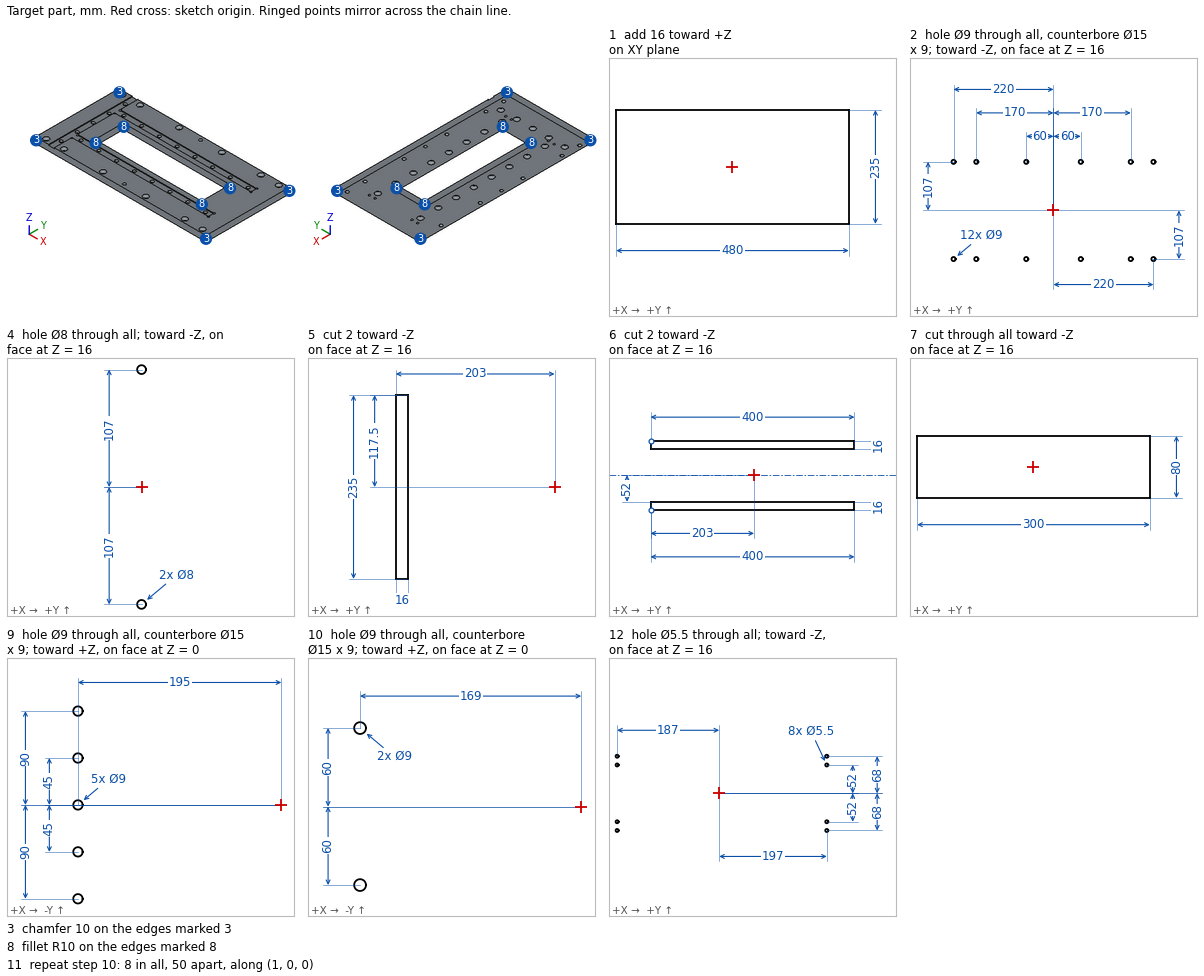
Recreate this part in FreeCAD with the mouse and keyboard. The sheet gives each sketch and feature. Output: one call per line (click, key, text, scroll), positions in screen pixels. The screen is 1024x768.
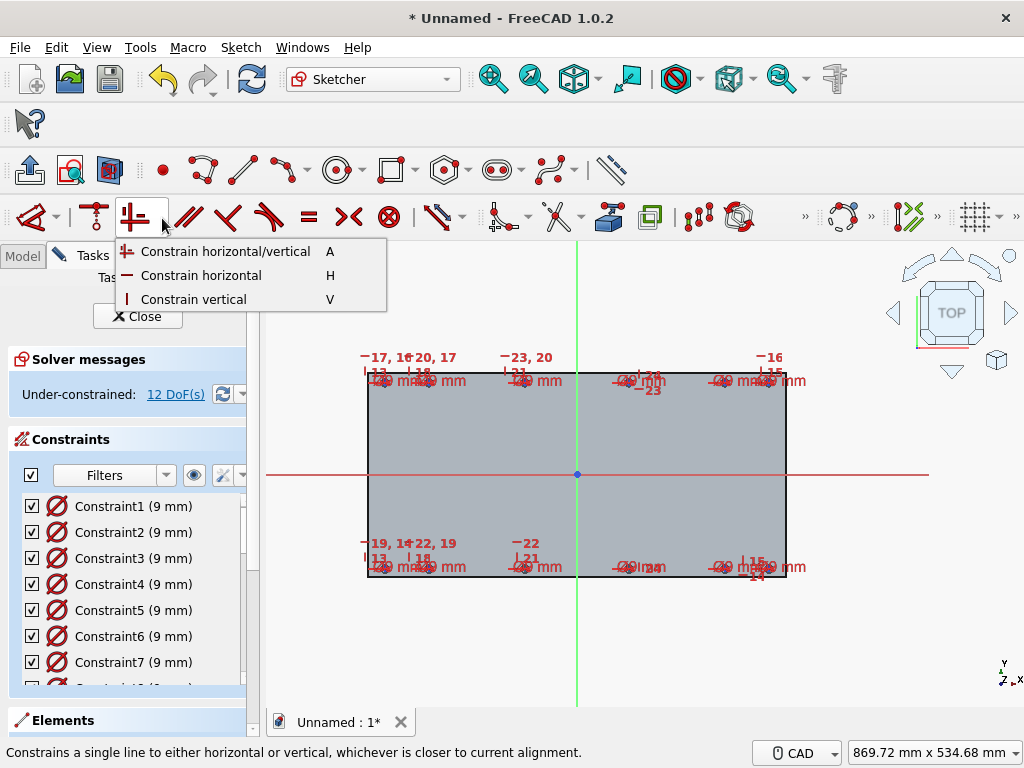
click(251, 275)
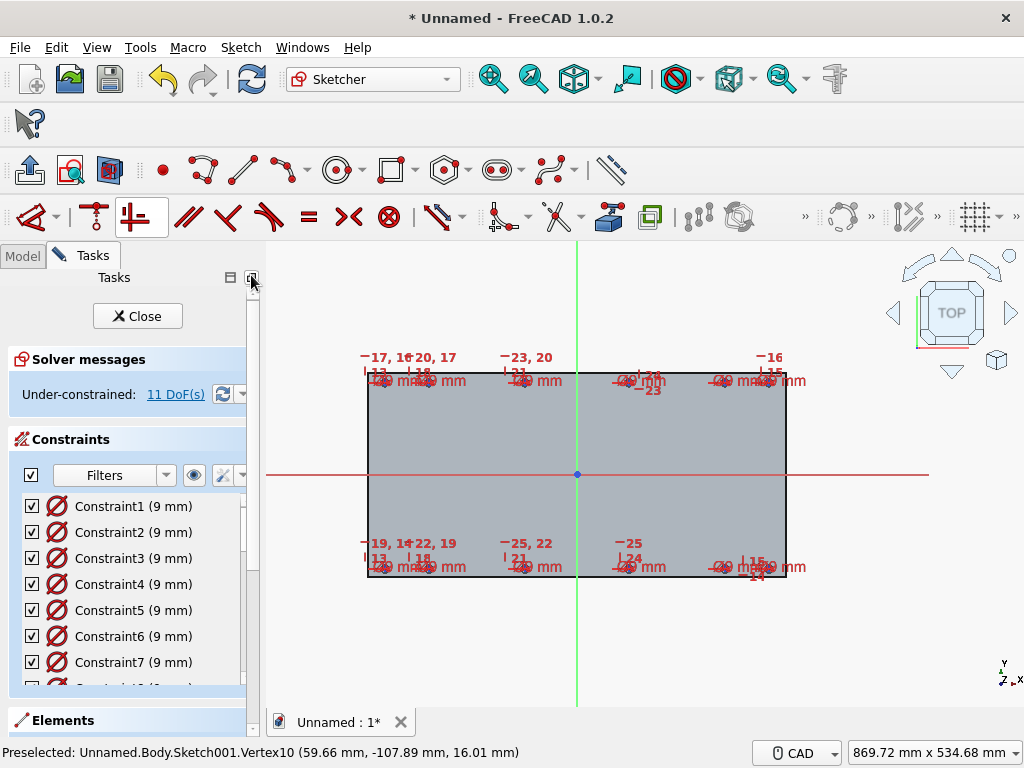
click(769, 383)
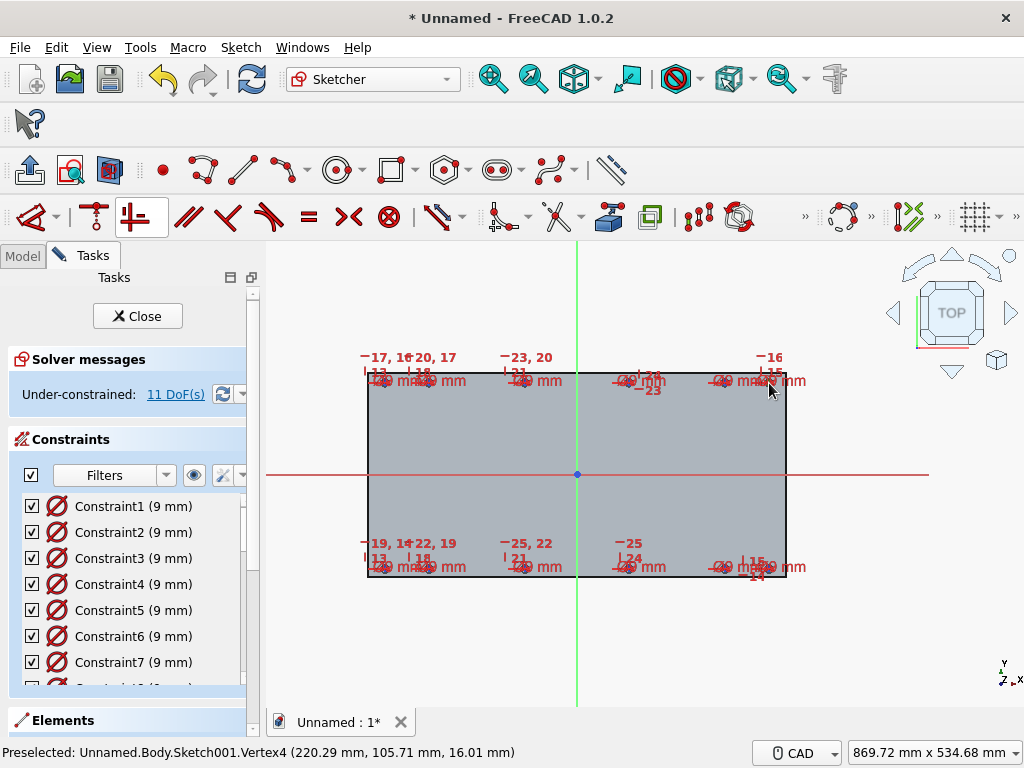
click(725, 383)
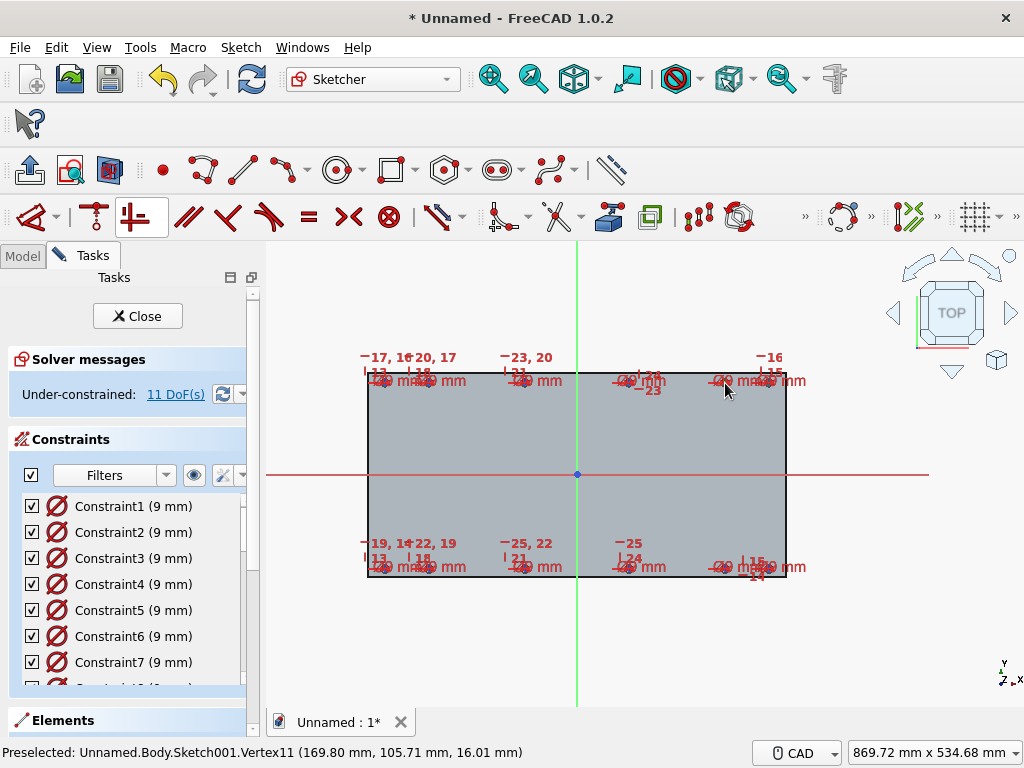
click(162, 218)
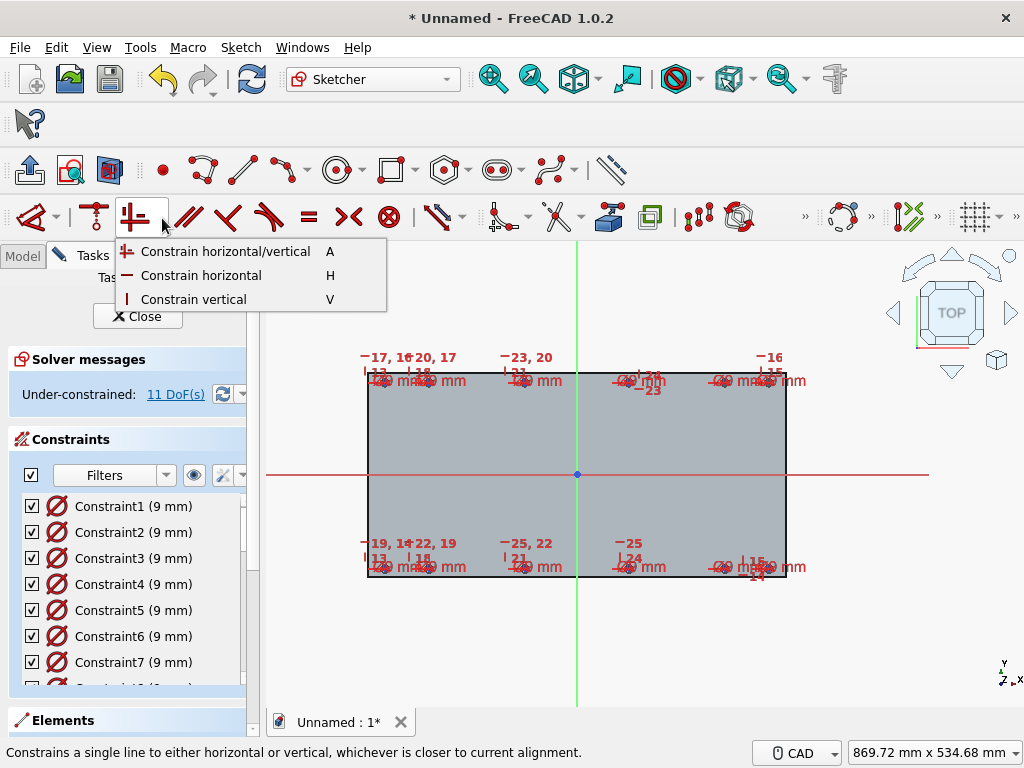
click(251, 275)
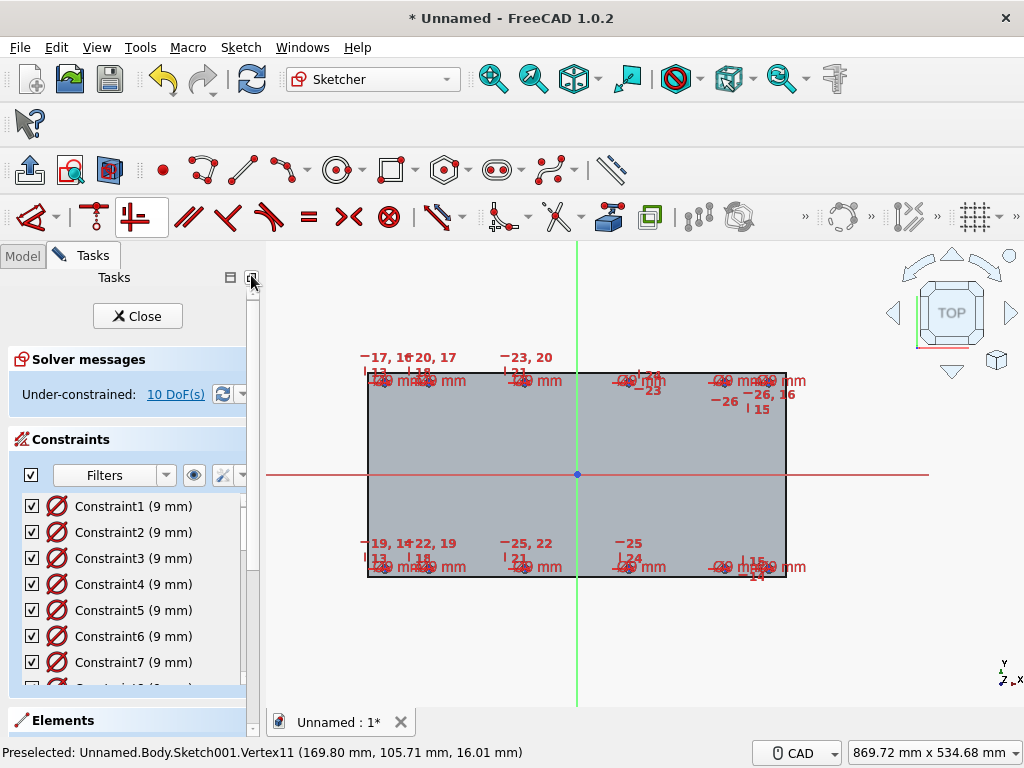
click(725, 383)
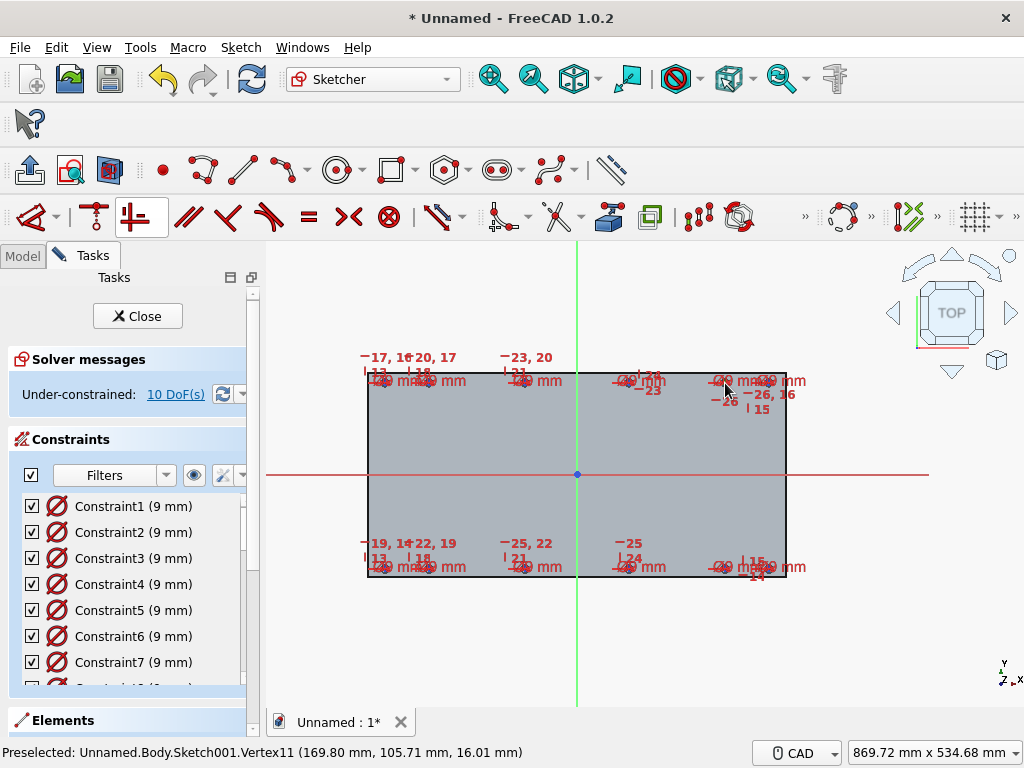
click(725, 569)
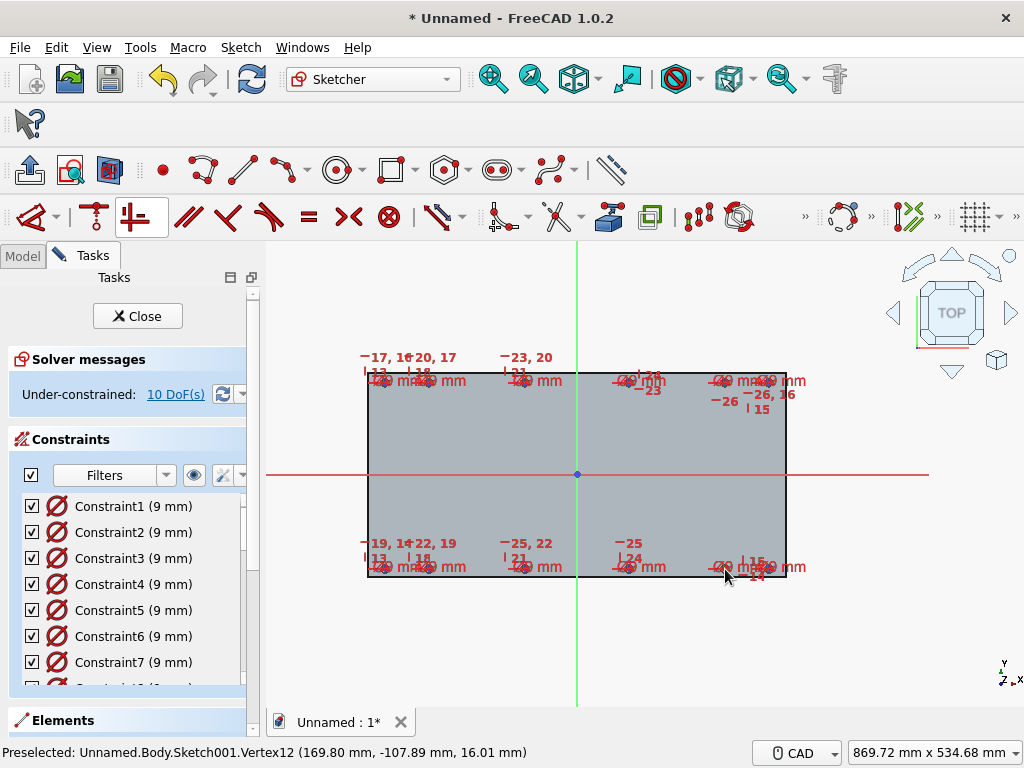
click(162, 218)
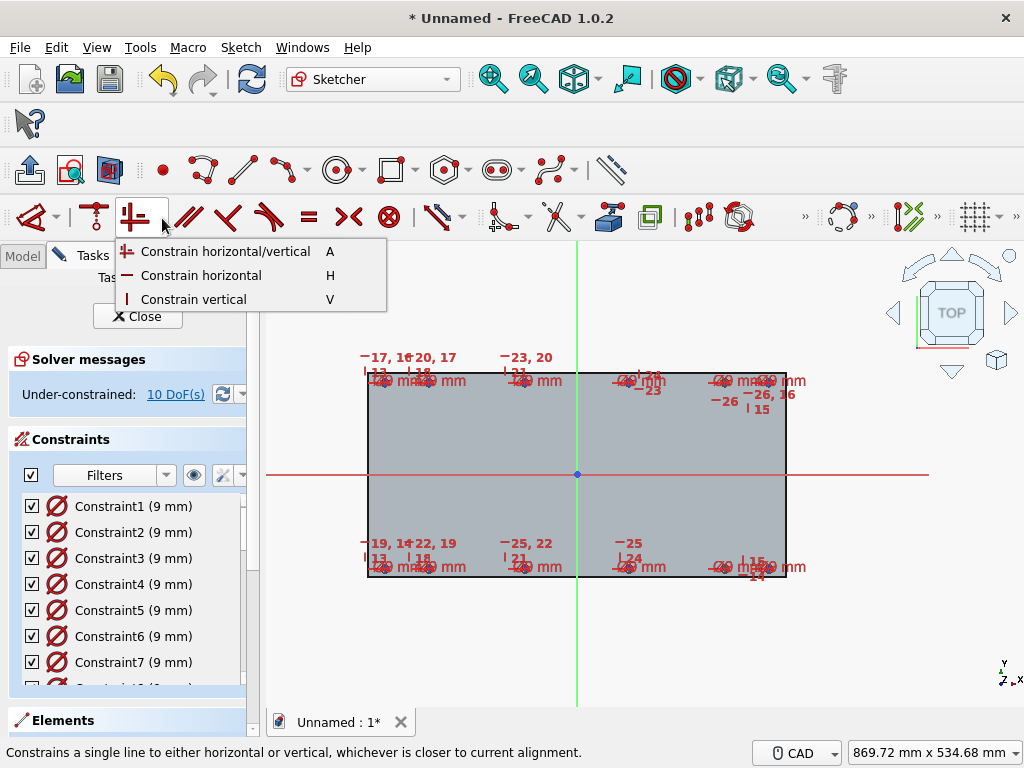
click(251, 299)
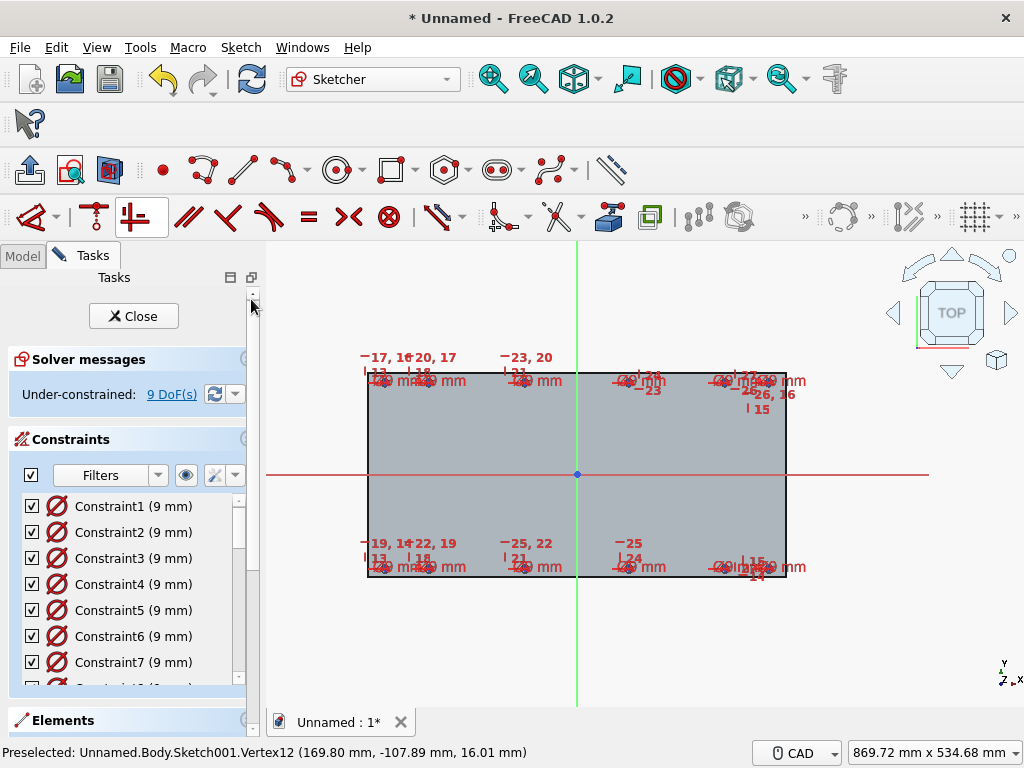
click(769, 569)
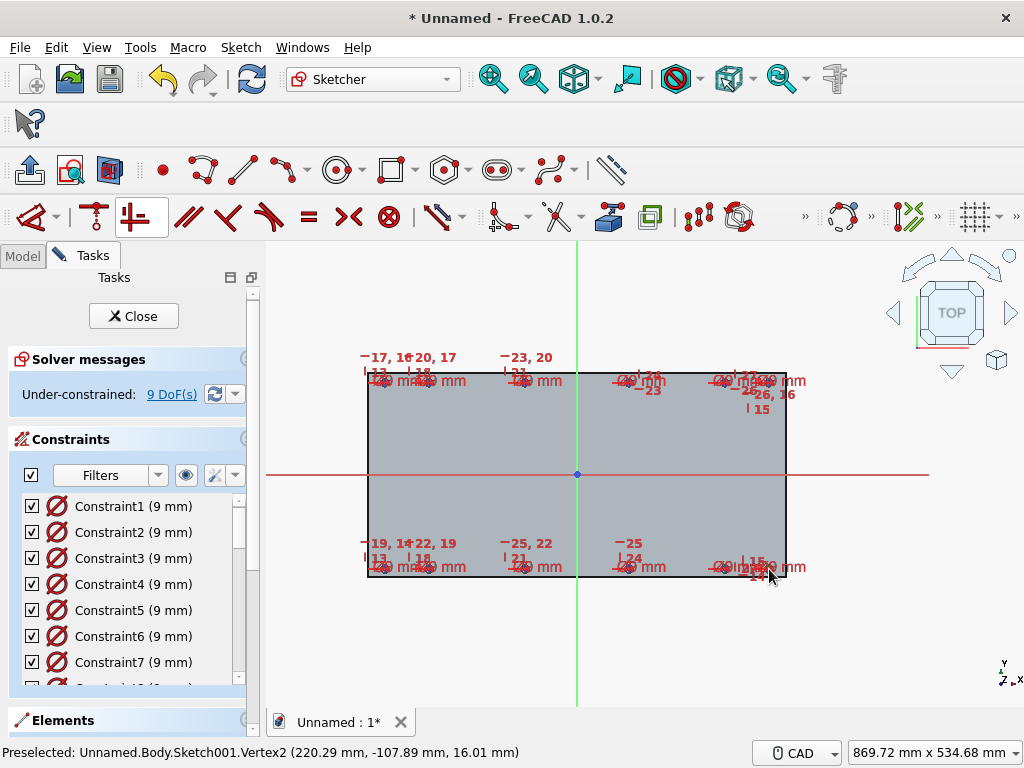
click(725, 569)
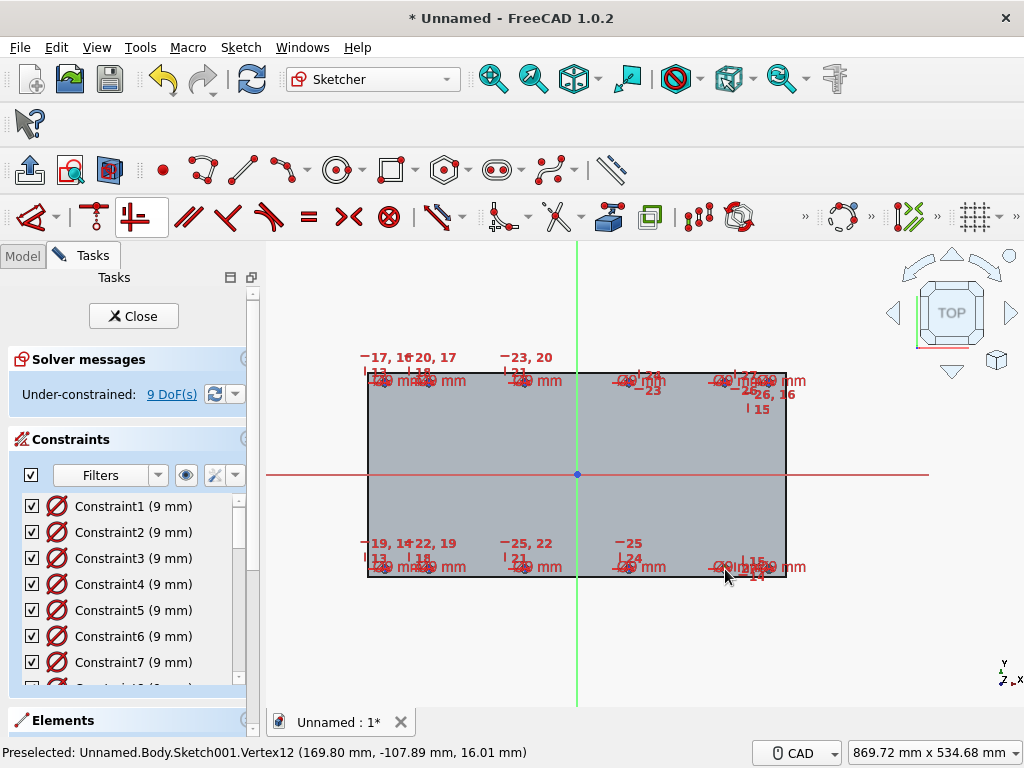
click(162, 218)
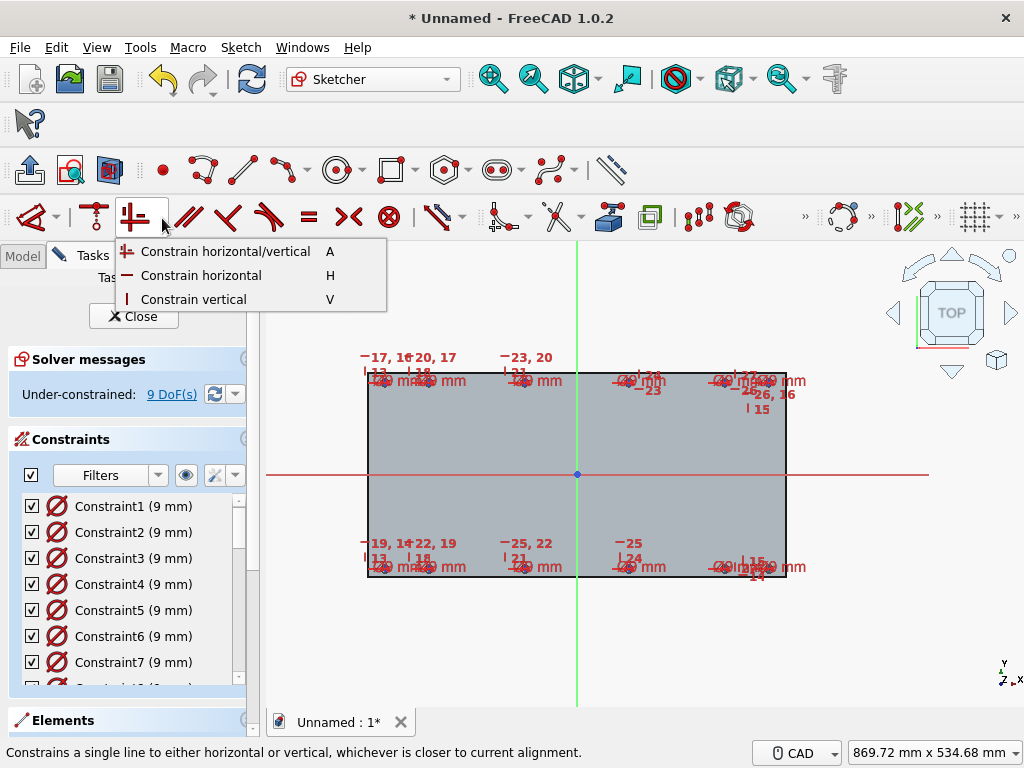
click(251, 275)